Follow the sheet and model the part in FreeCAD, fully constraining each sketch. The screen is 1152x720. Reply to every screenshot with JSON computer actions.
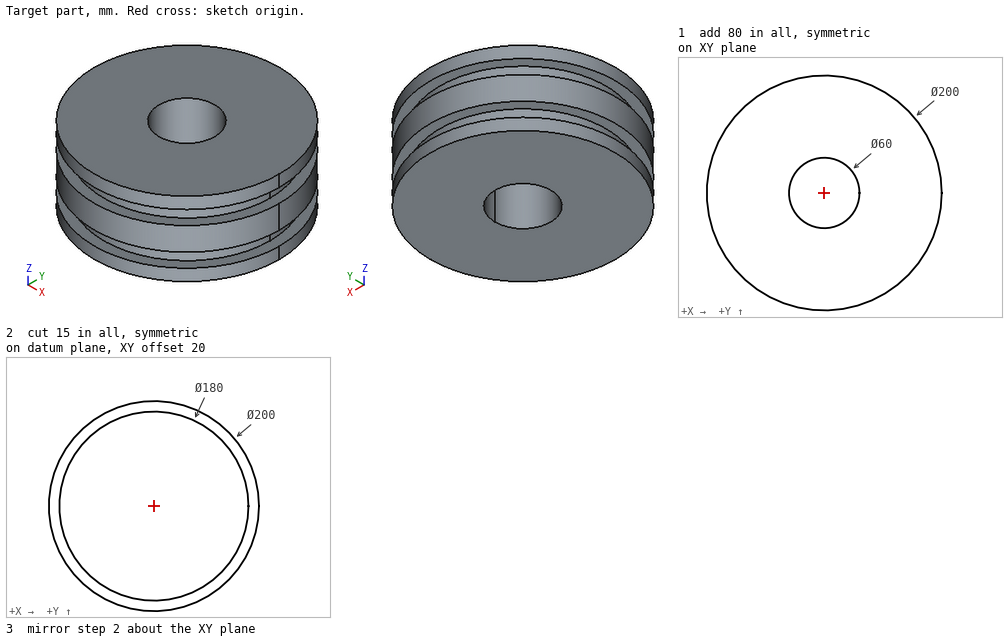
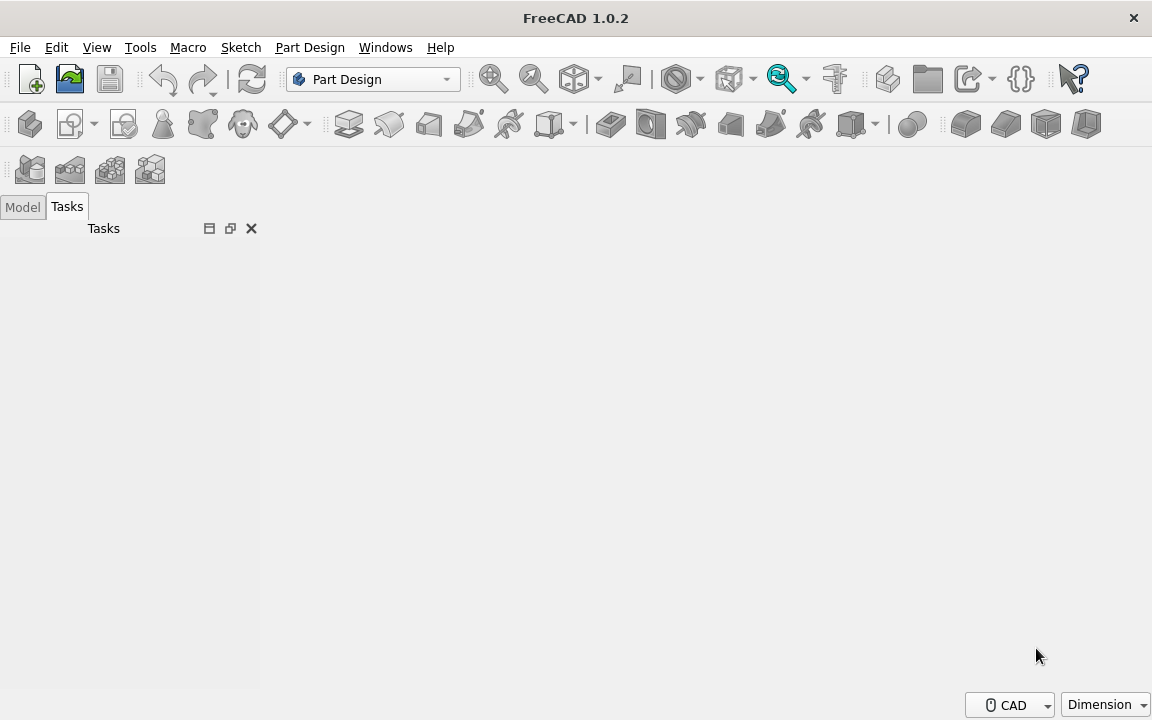
{"action": "left_click", "coordinate": [30, 80]}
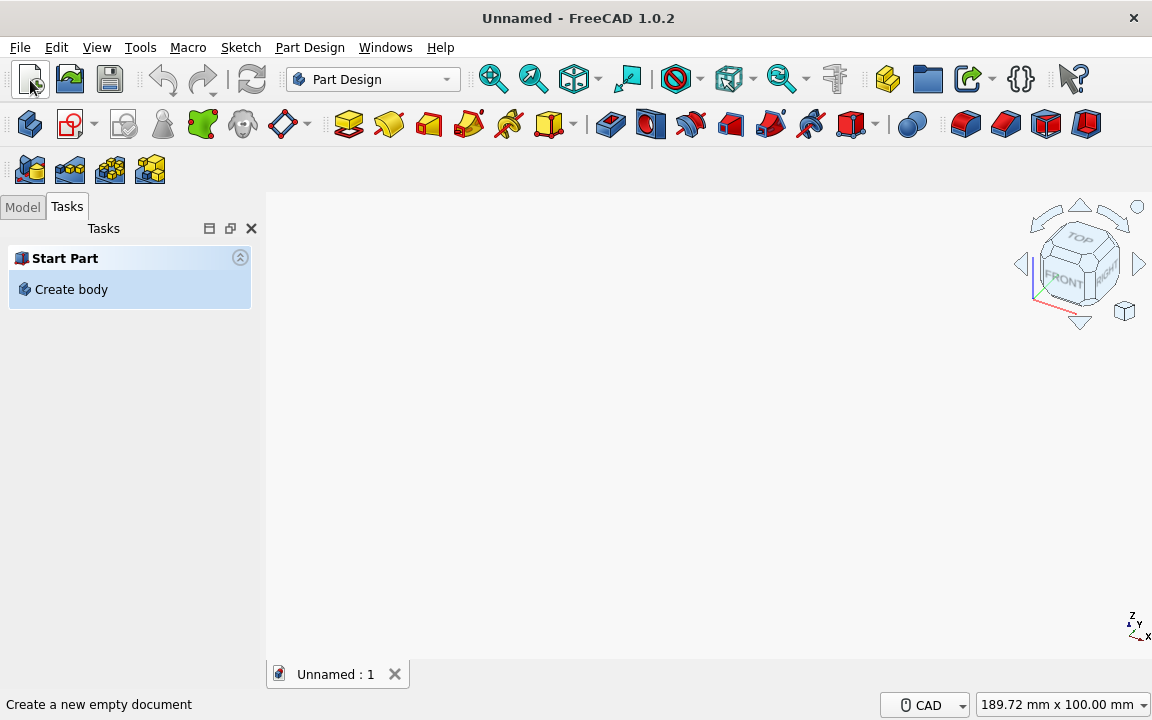
{"action": "left_click", "coordinate": [70, 124]}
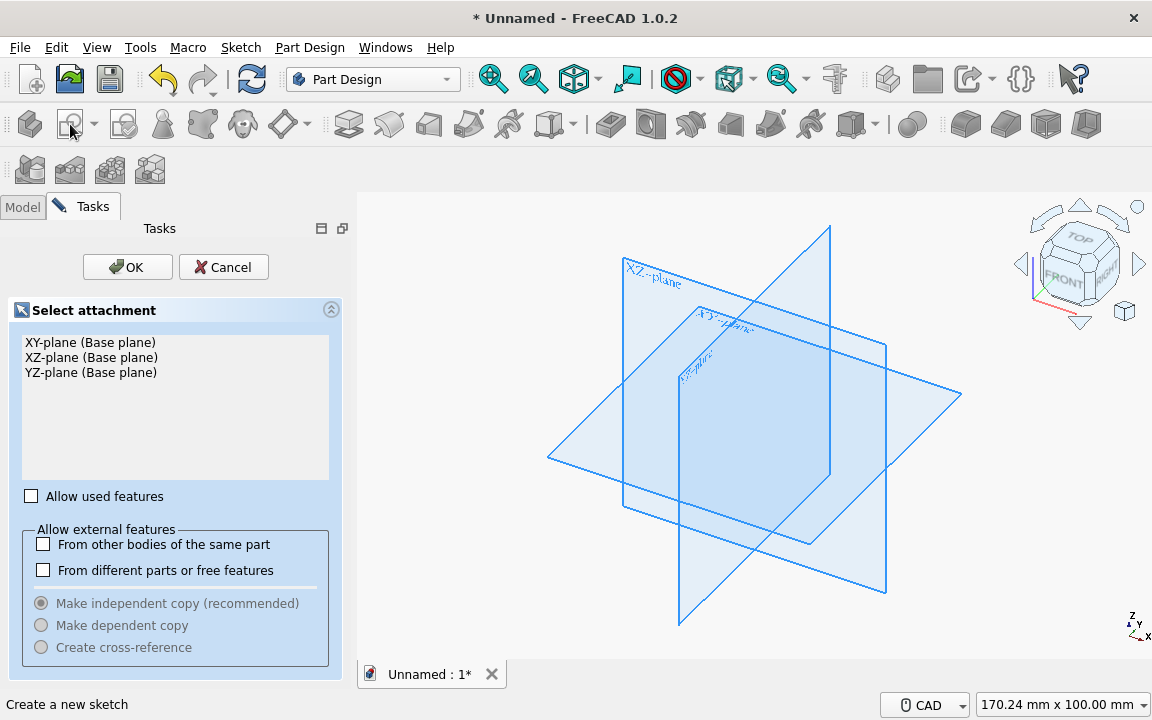
{"action": "left_click", "coordinate": [82, 342]}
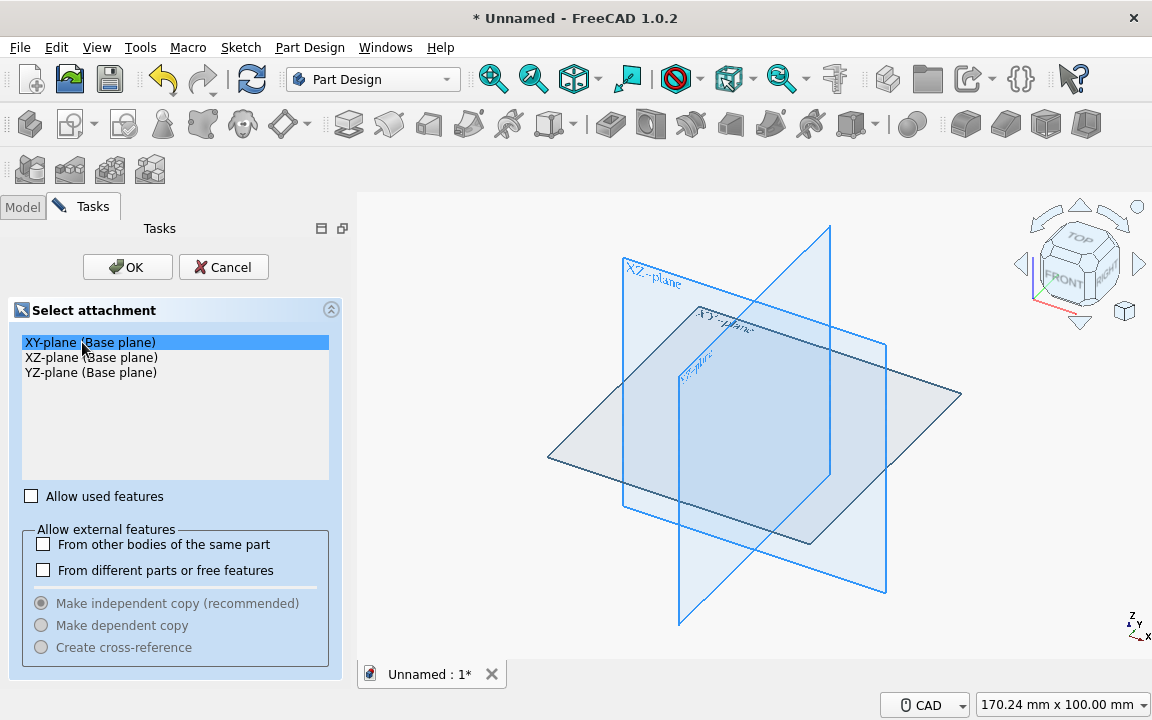
{"action": "left_click", "coordinate": [128, 267]}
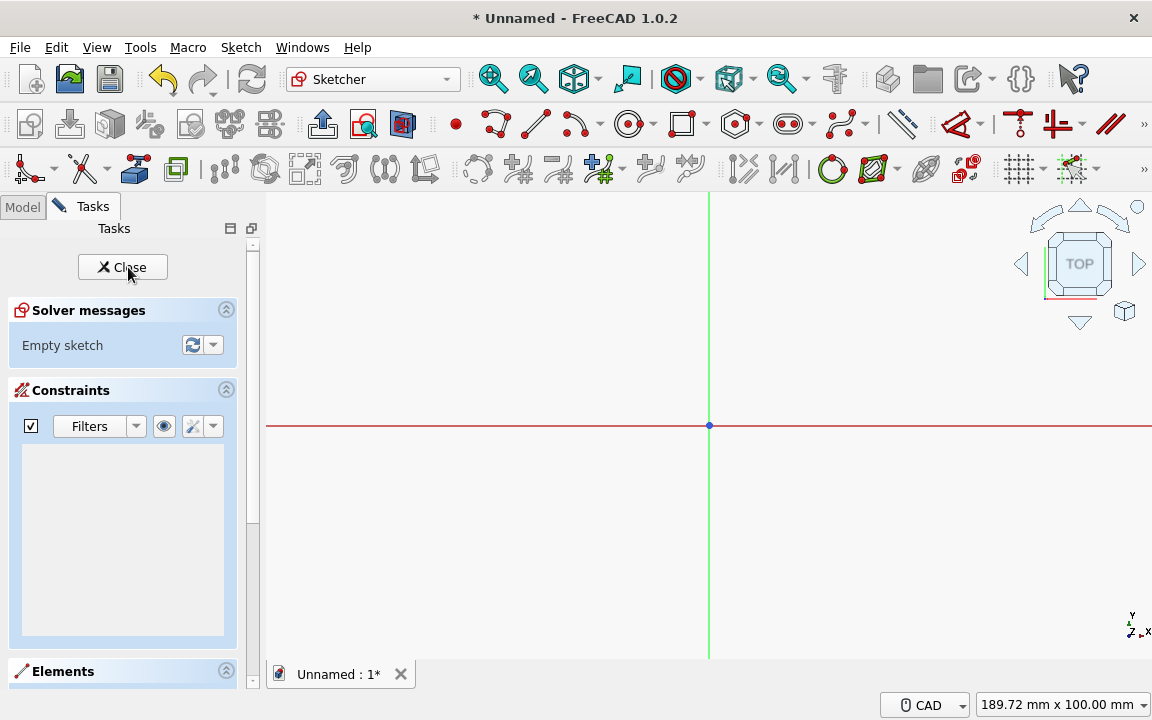
{"action": "scroll", "coordinate": [611, 426], "scroll_direction": "down", "scroll_amount": 6}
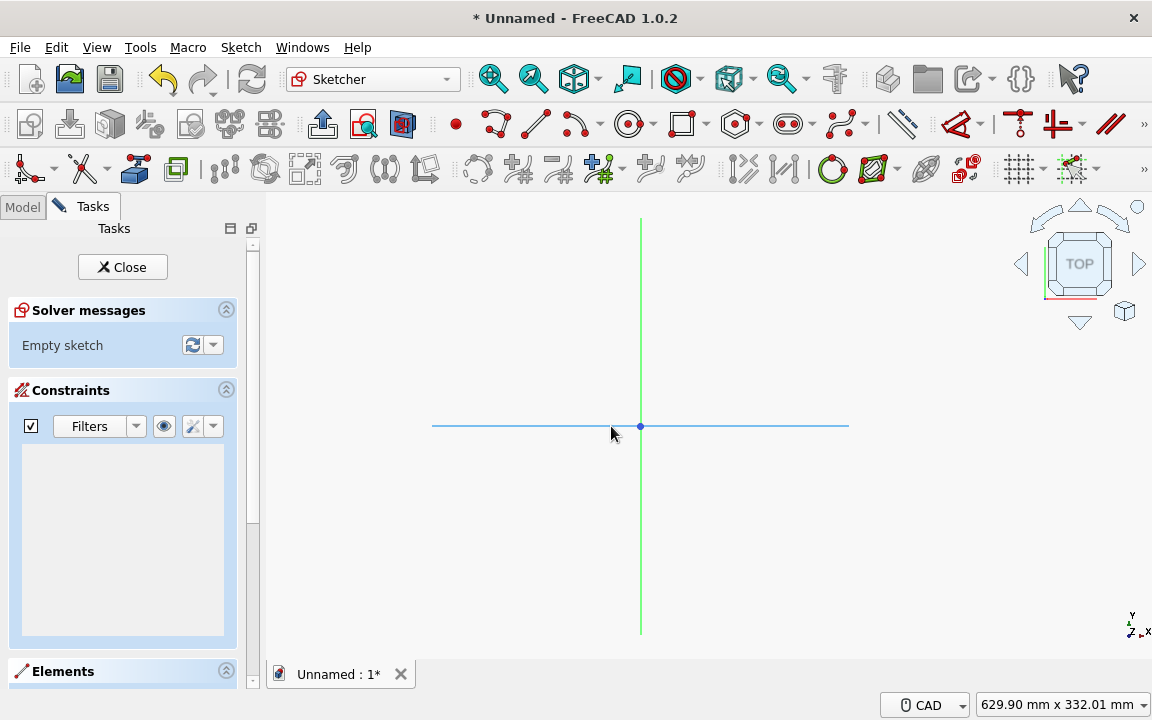
{"action": "left_click", "coordinate": [630, 124]}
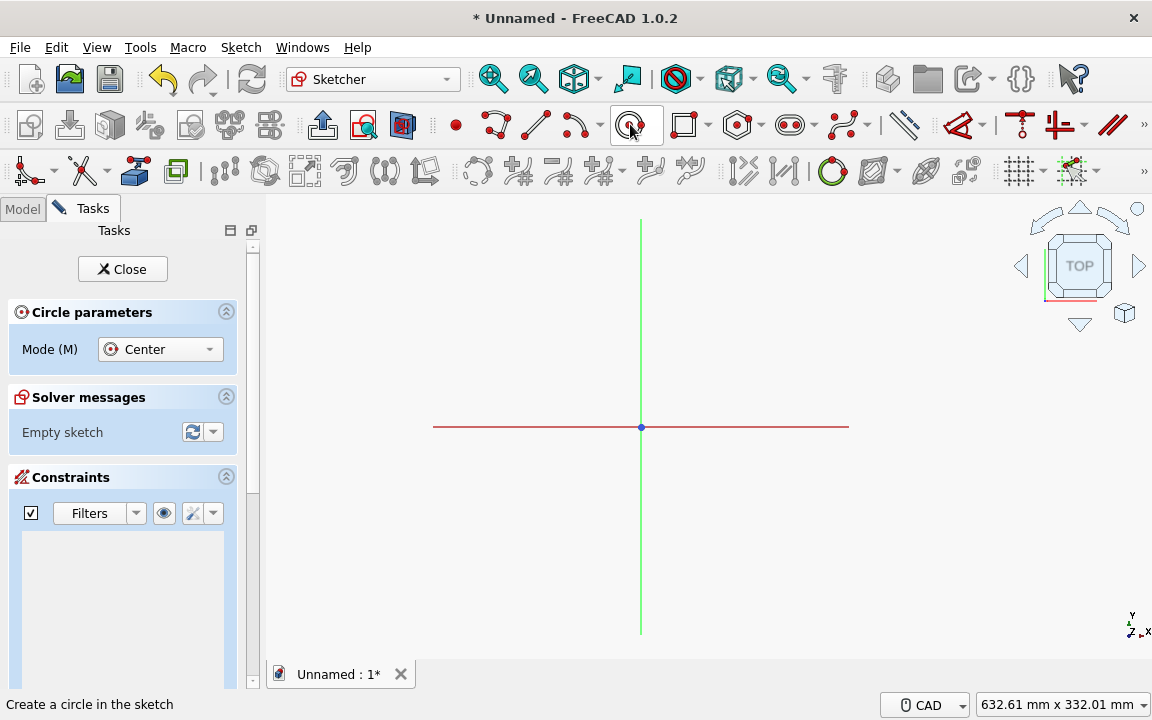
{"action": "left_click", "coordinate": [641, 427]}
{"action": "left_click", "coordinate": [740, 328]}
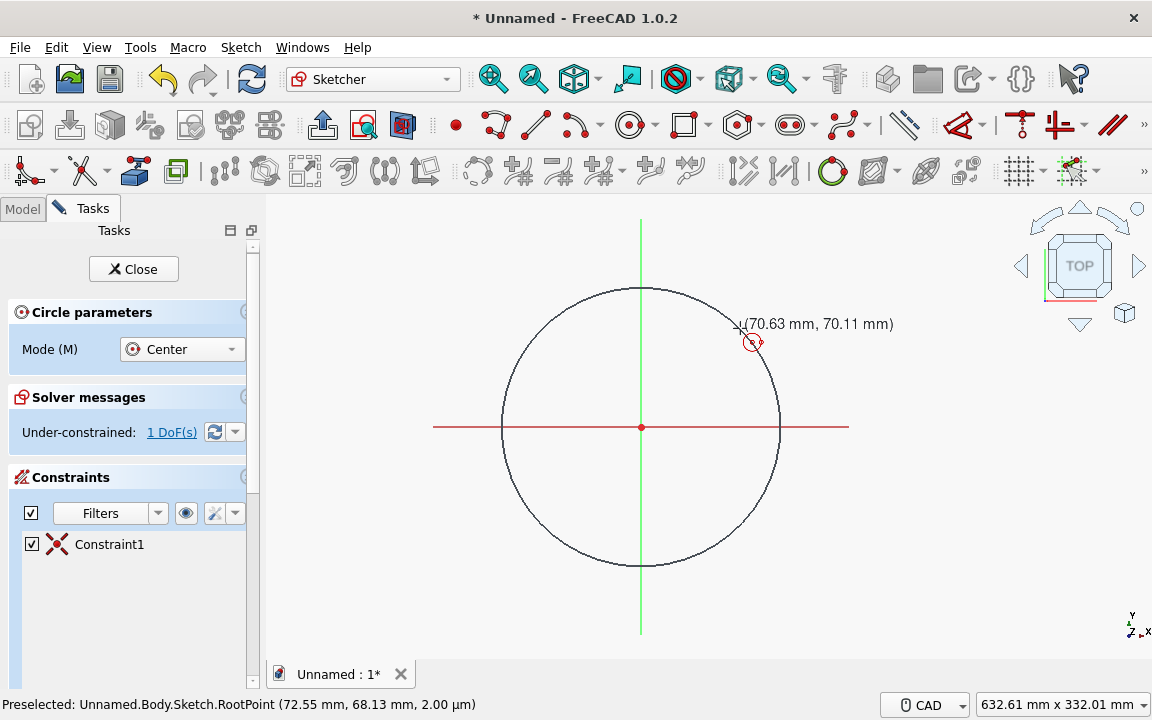
{"action": "left_click", "coordinate": [641, 427]}
{"action": "left_click", "coordinate": [671, 397]}
{"action": "key", "text": "Escape"}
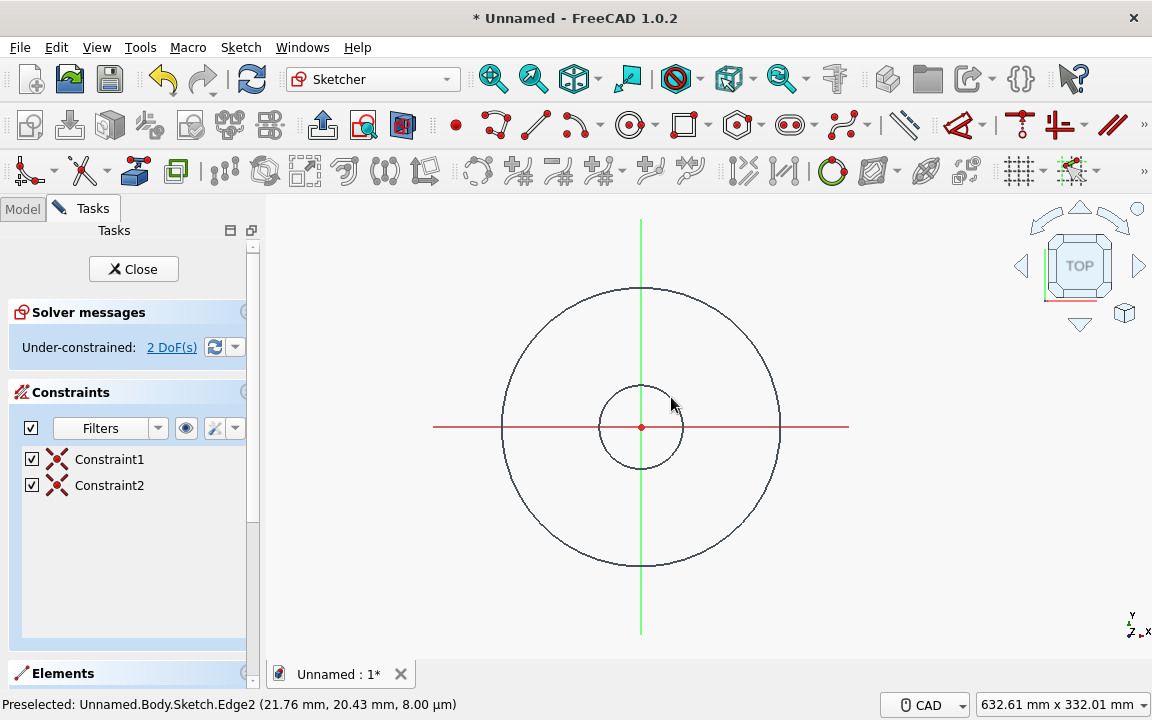
{"action": "left_click", "coordinate": [958, 126]}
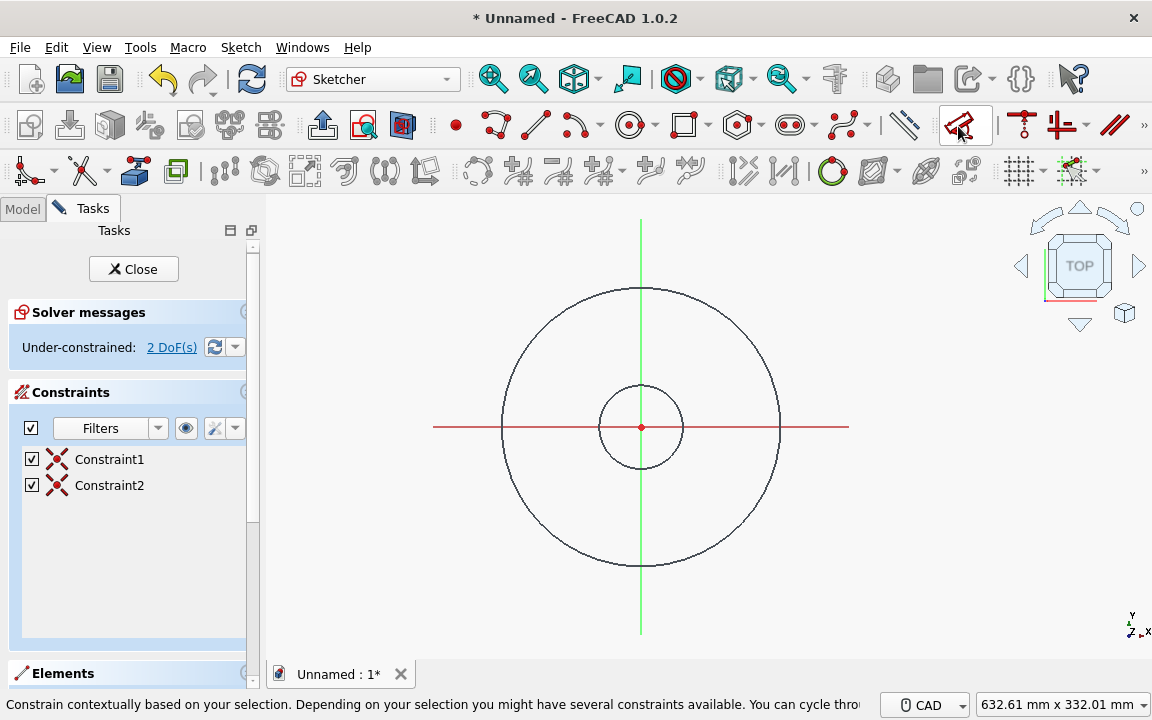
{"action": "left_click", "coordinate": [739, 328]}
{"action": "left_click", "coordinate": [761, 305]}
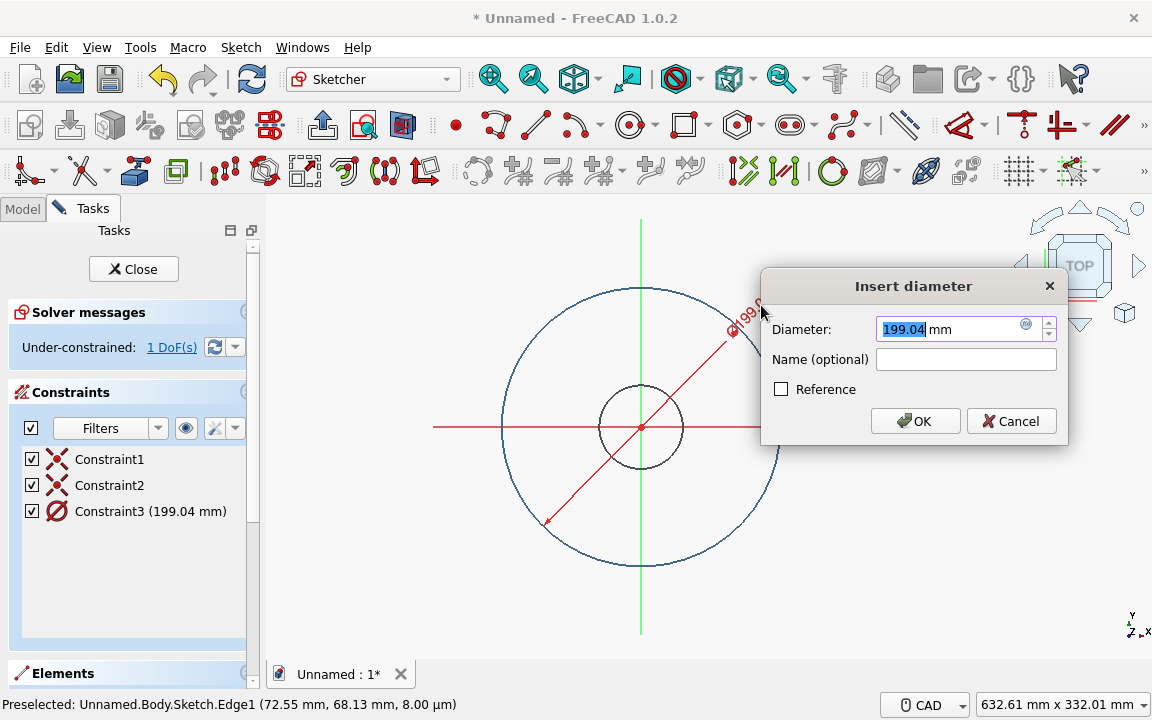
{"action": "type", "text": "200"}
{"action": "key", "text": "Return"}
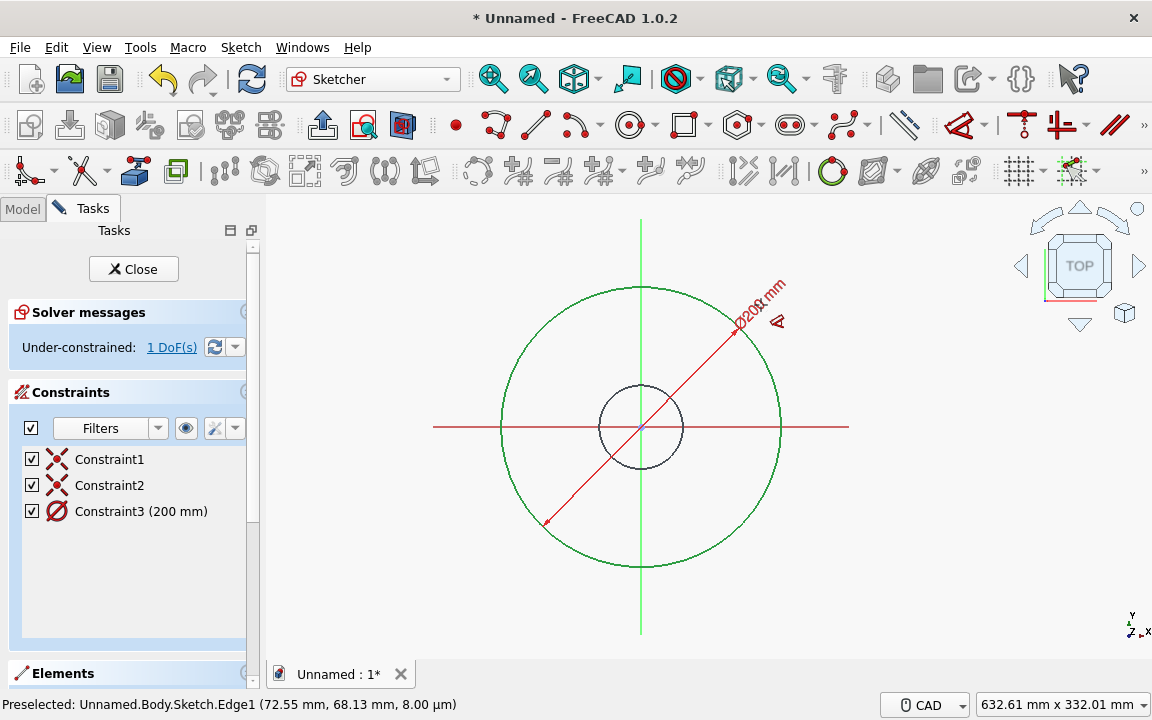
{"action": "left_click", "coordinate": [671, 398]}
{"action": "left_click", "coordinate": [694, 376]}